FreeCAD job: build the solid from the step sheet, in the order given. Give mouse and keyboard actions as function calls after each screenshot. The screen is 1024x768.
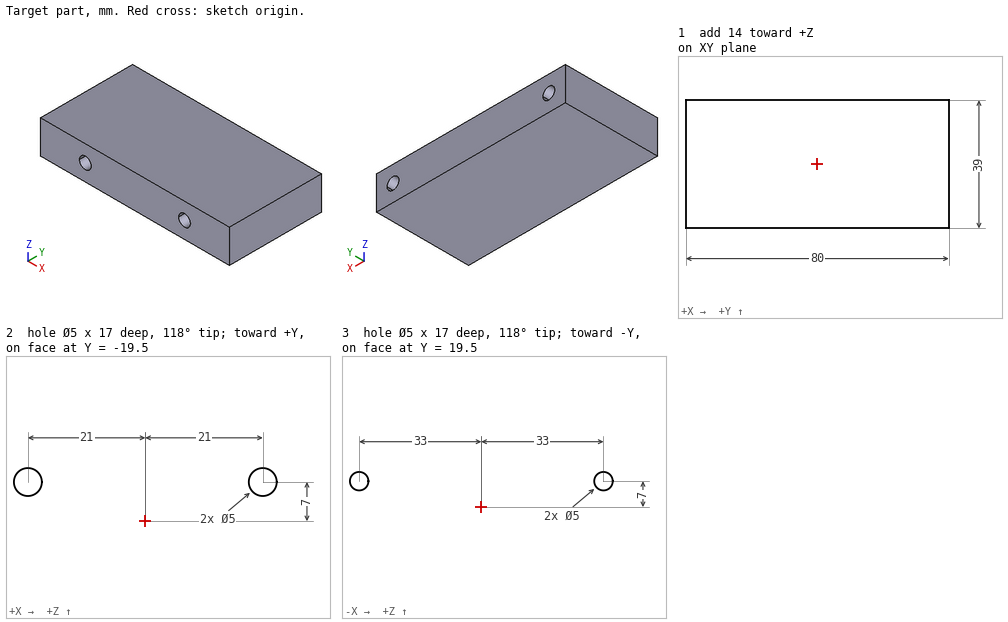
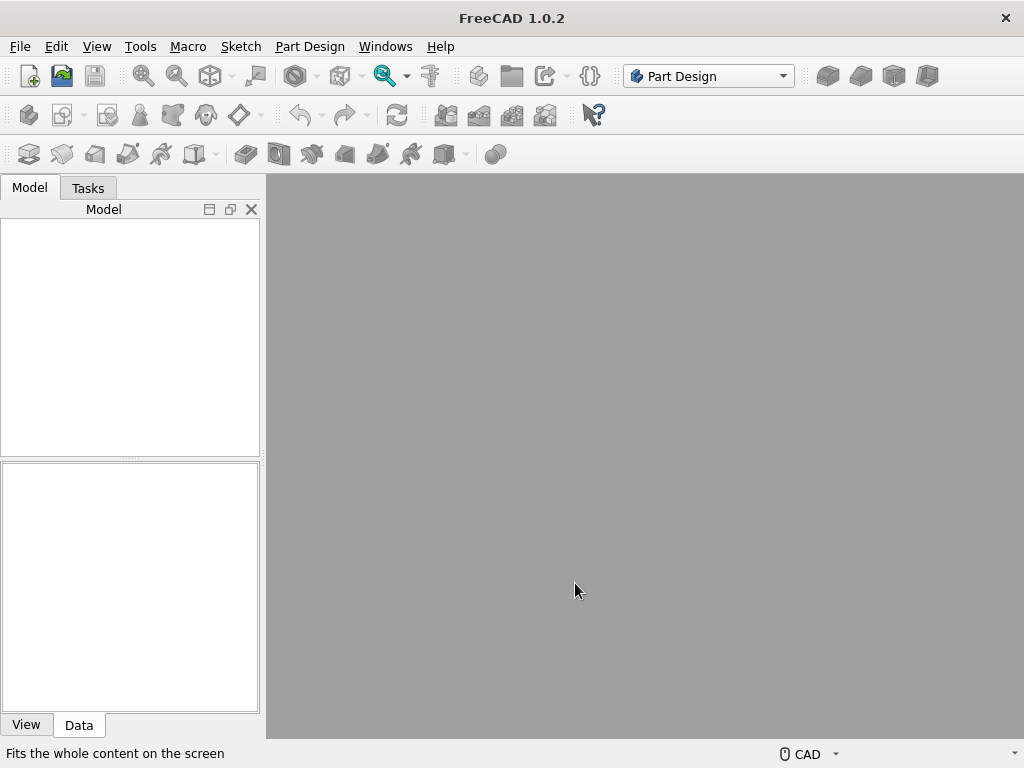
click(29, 76)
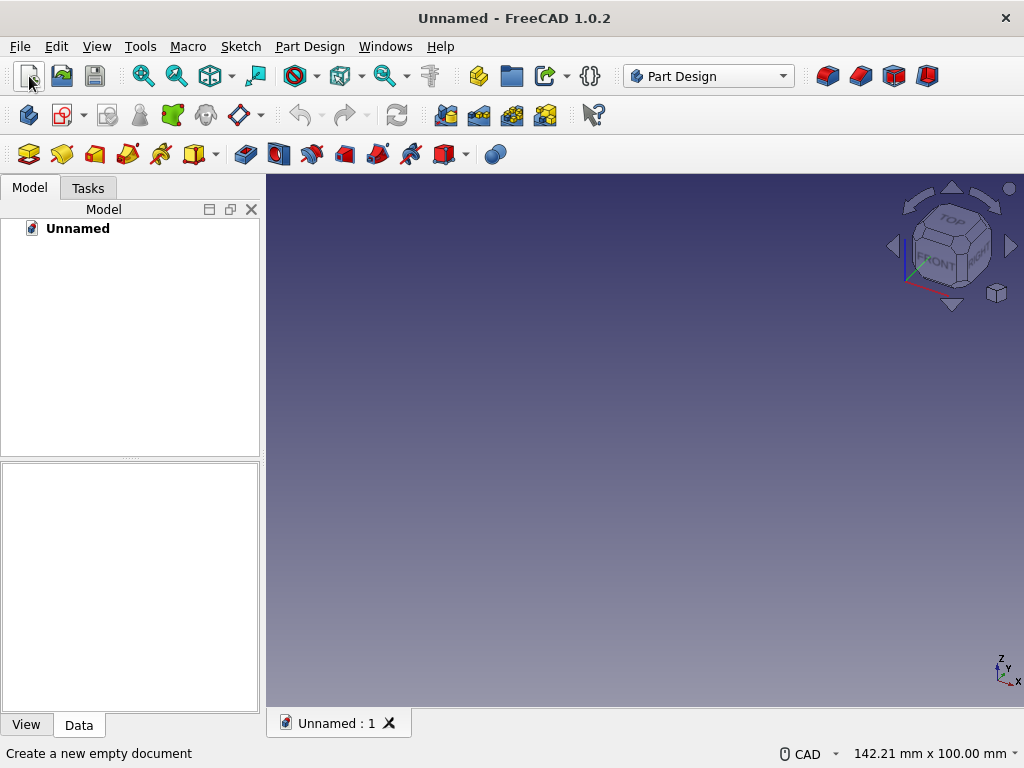
click(62, 116)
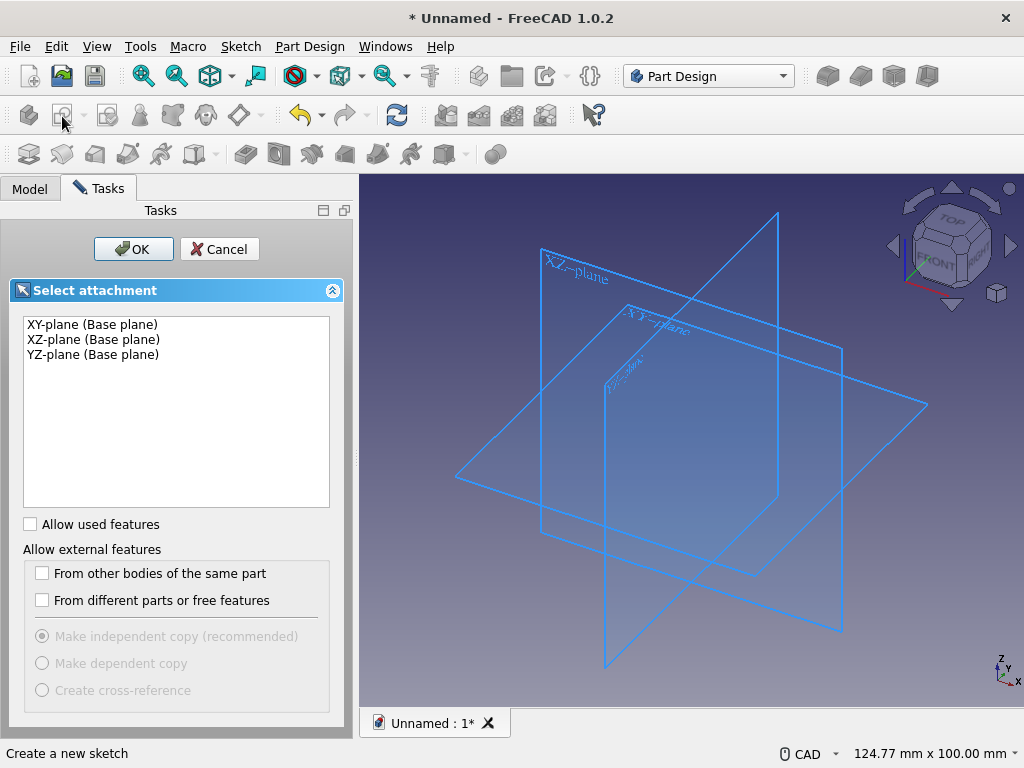
click(84, 324)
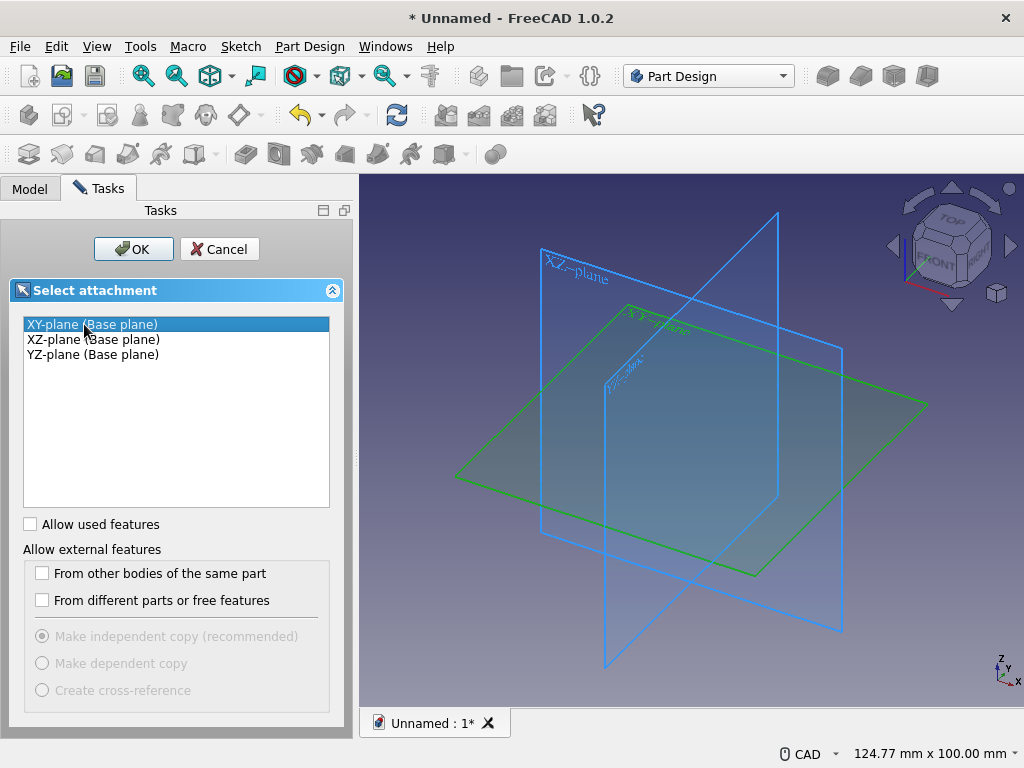
click(134, 249)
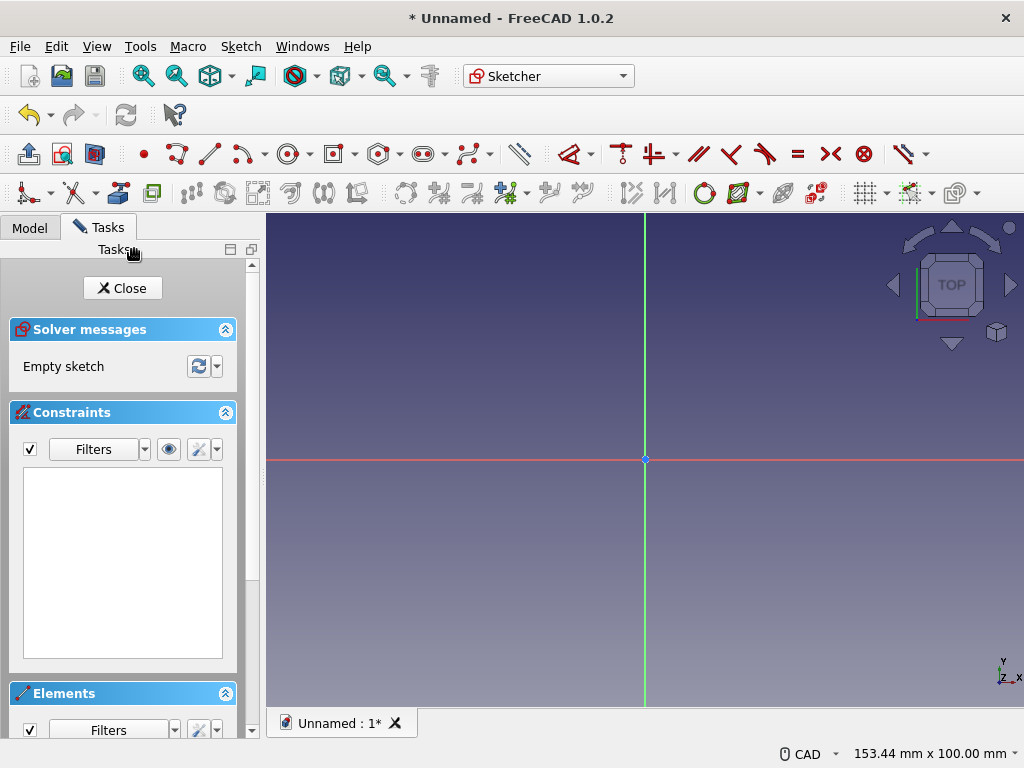
scroll(294, 460, down, 1)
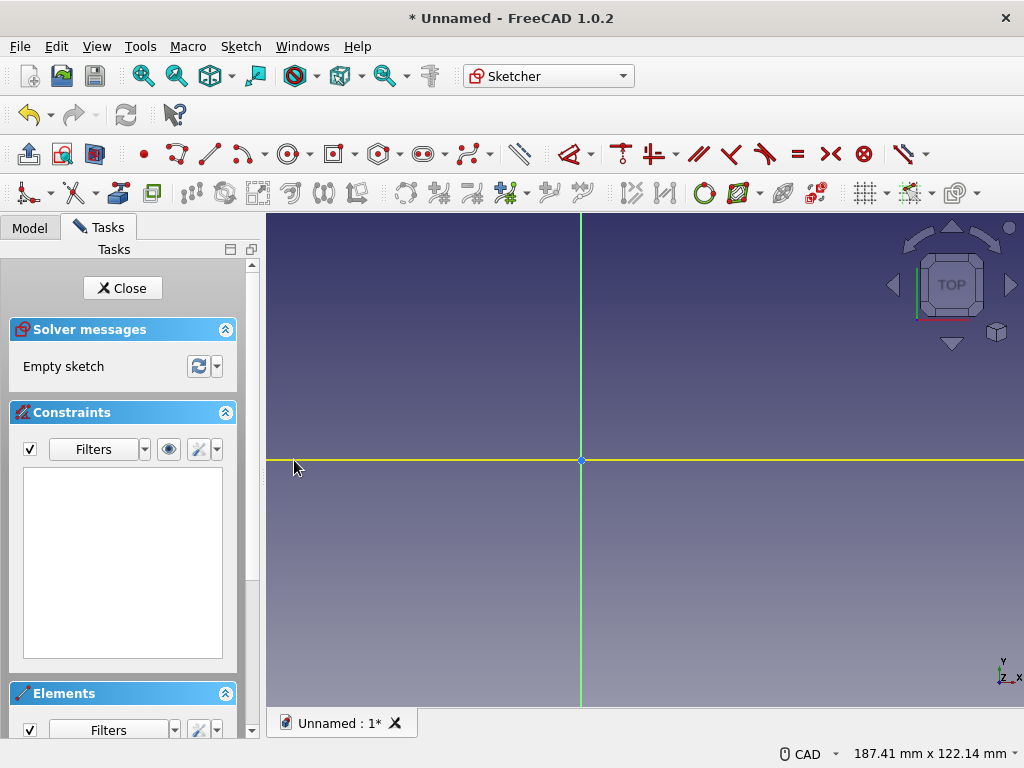
click(332, 154)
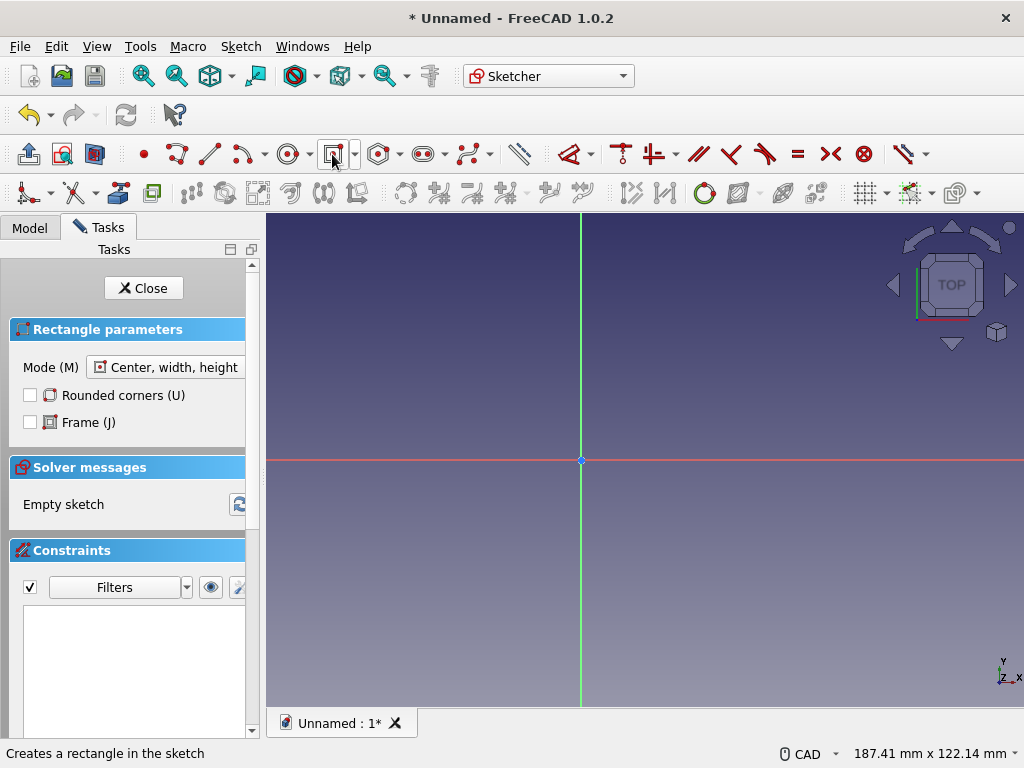
click(581, 460)
move(743, 381)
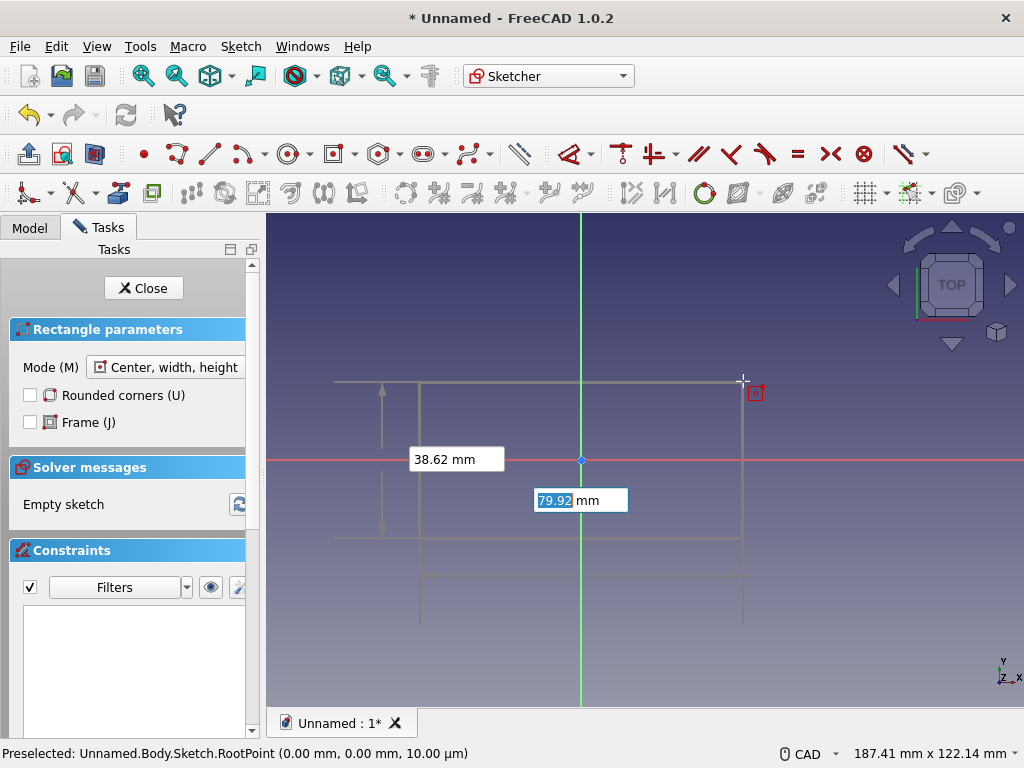
text(80)
key(Tab)
text(39)
key(Return)
key(Escape)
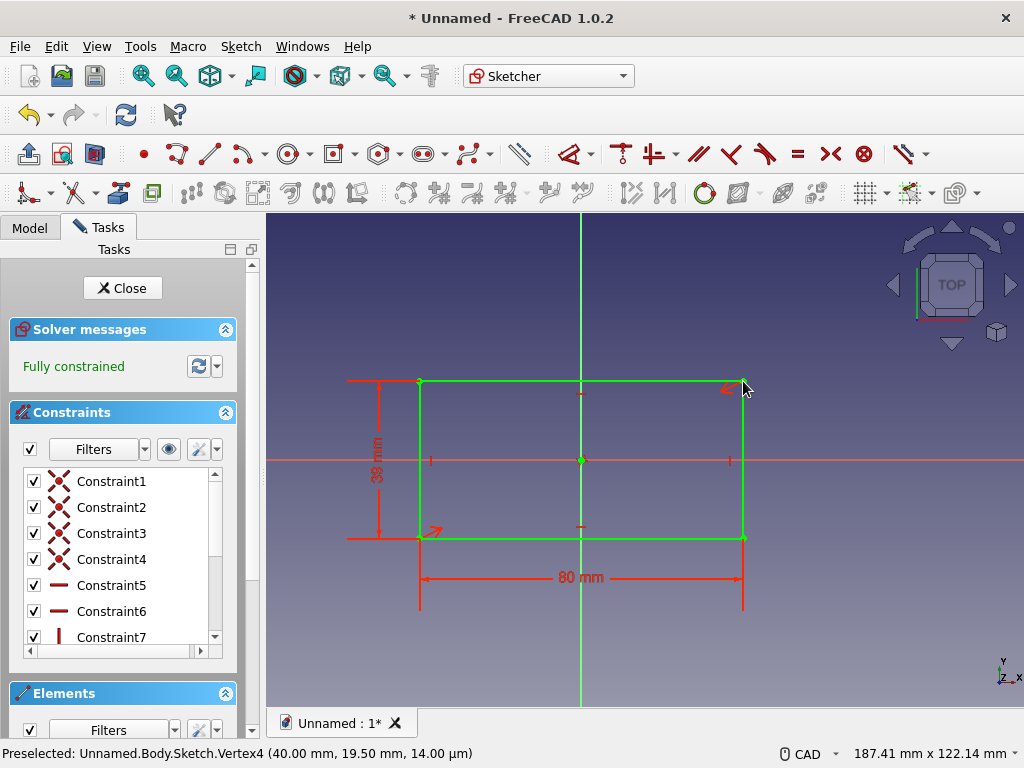
click(123, 288)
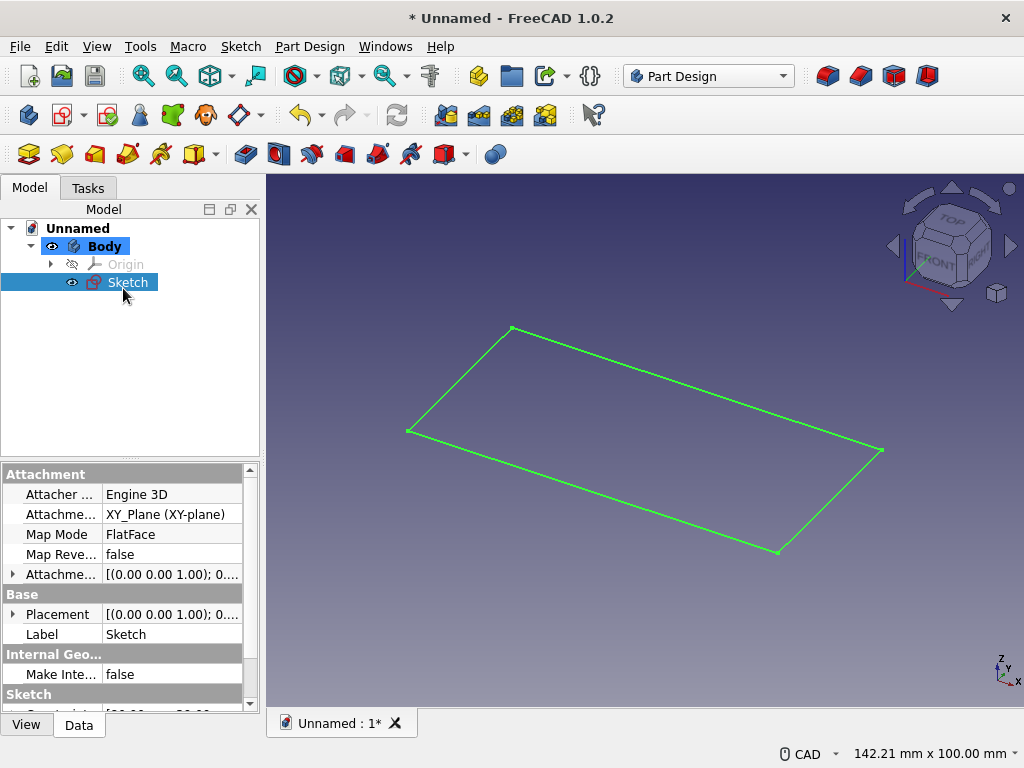
click(29, 154)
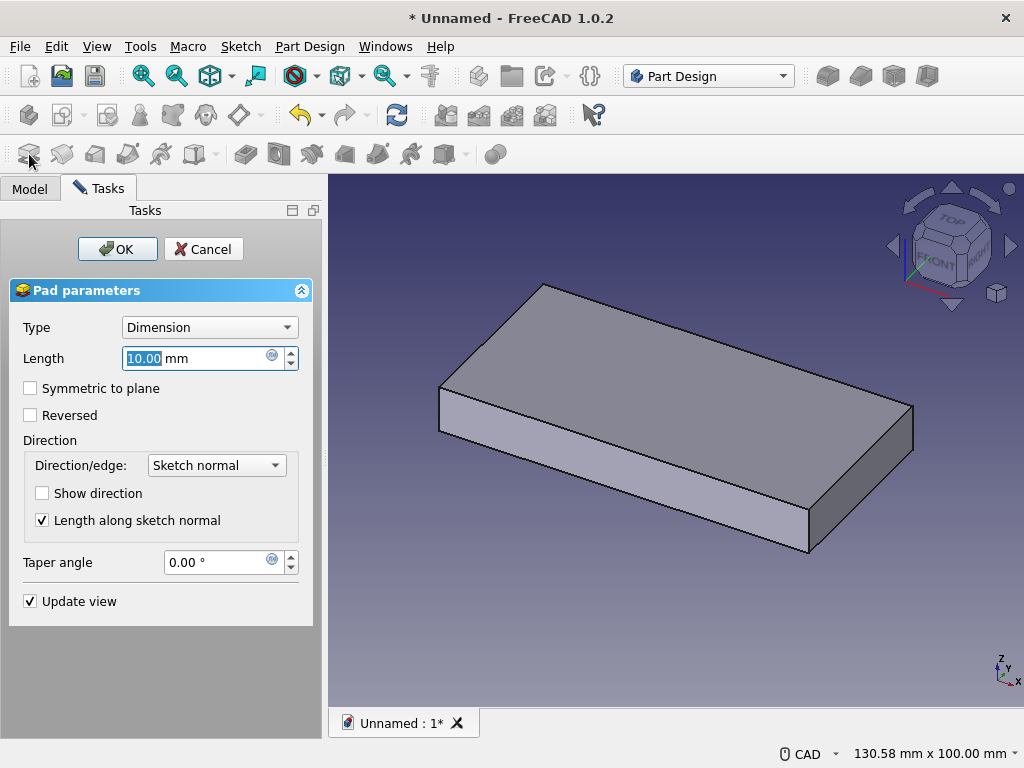
text(14)
key(Tab)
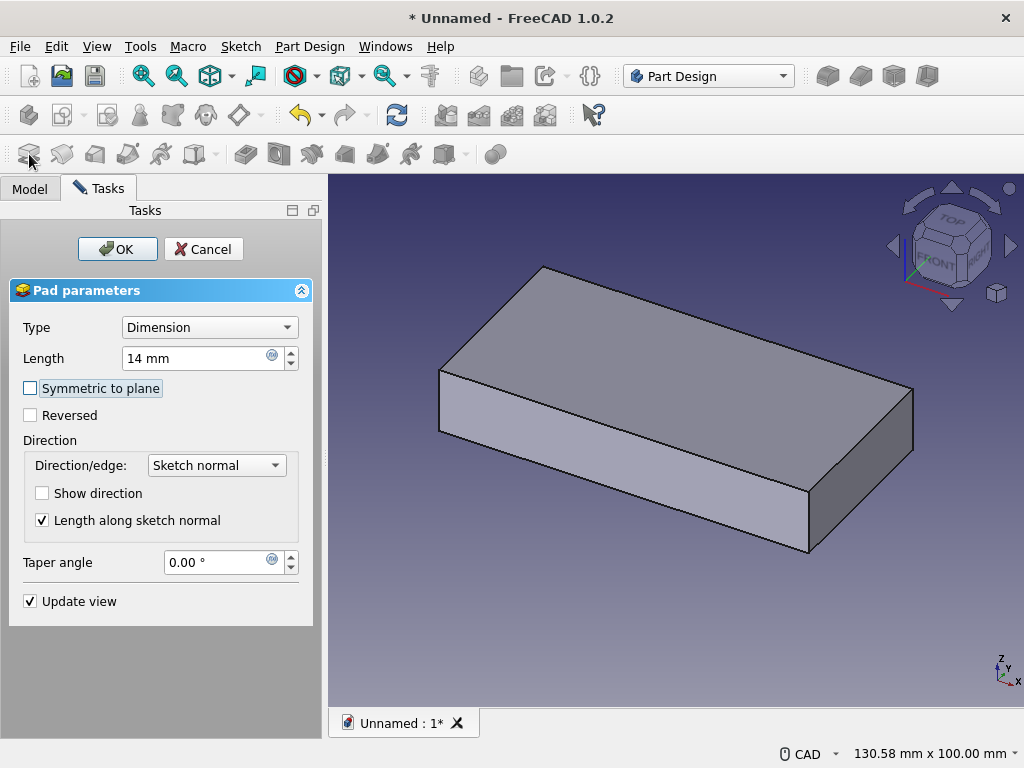
click(118, 249)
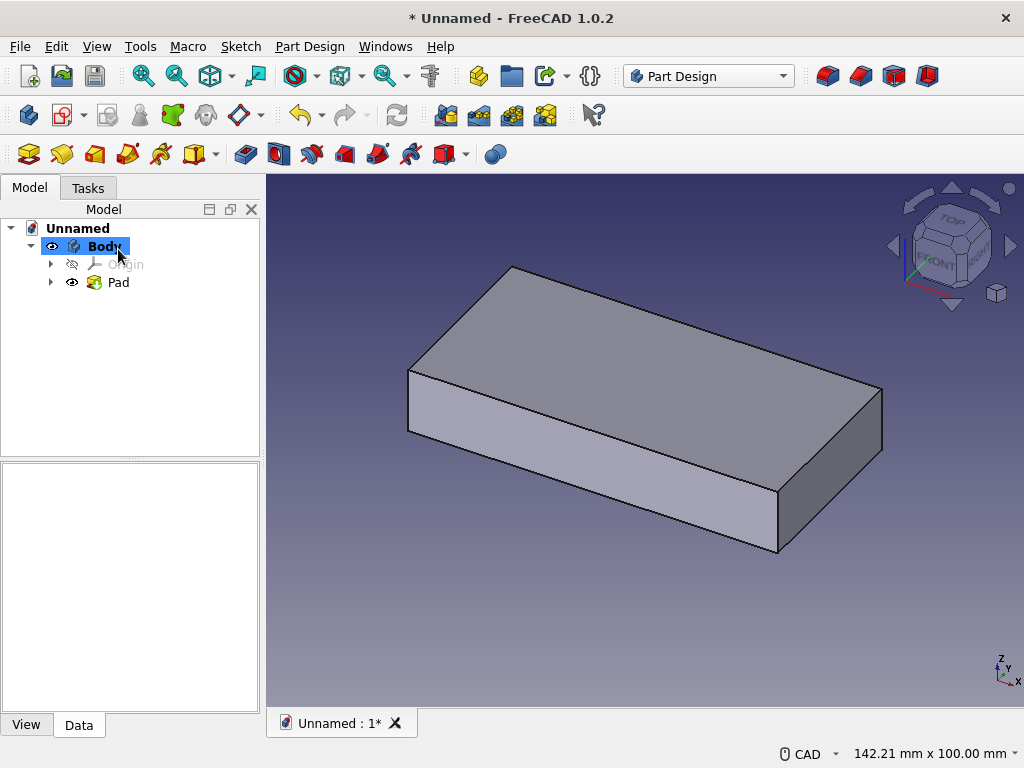
click(699, 496)